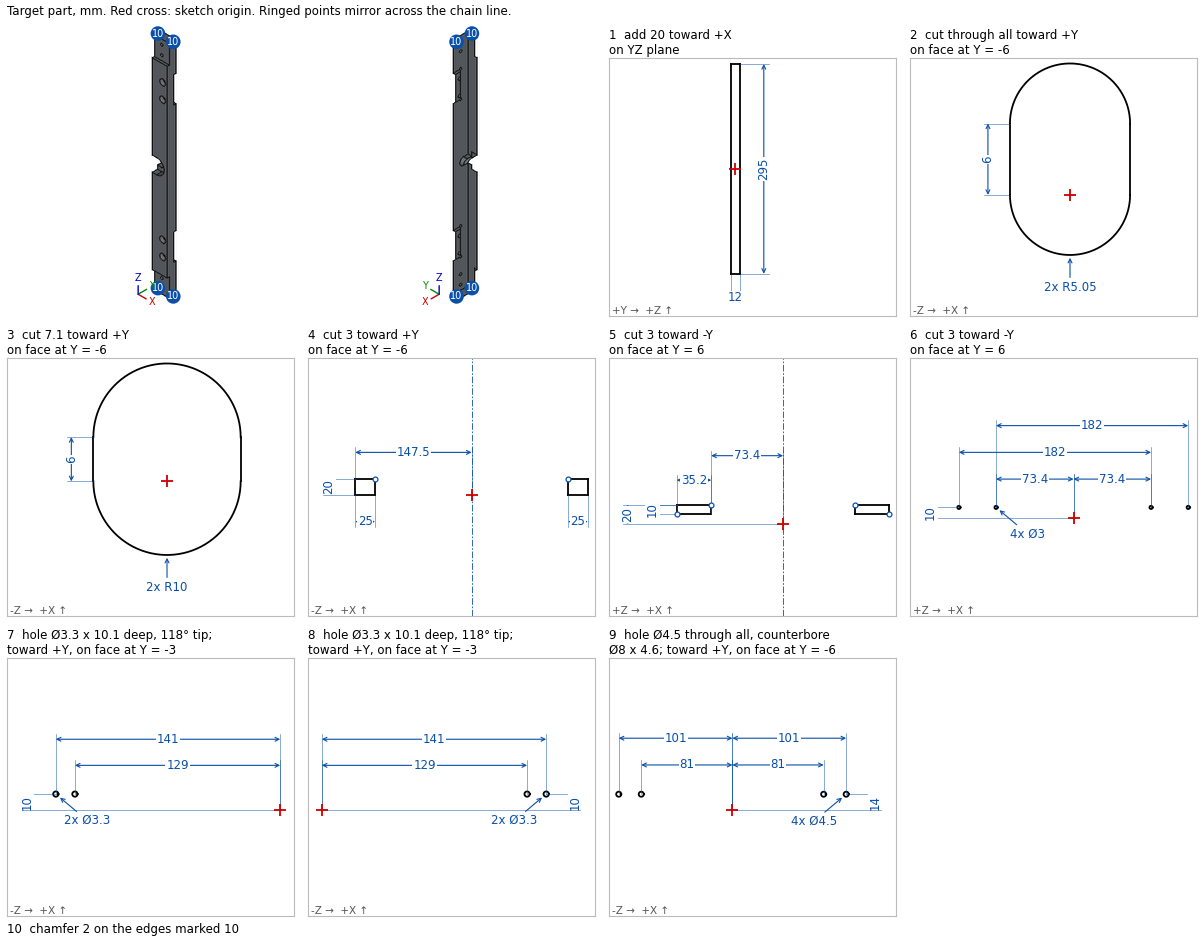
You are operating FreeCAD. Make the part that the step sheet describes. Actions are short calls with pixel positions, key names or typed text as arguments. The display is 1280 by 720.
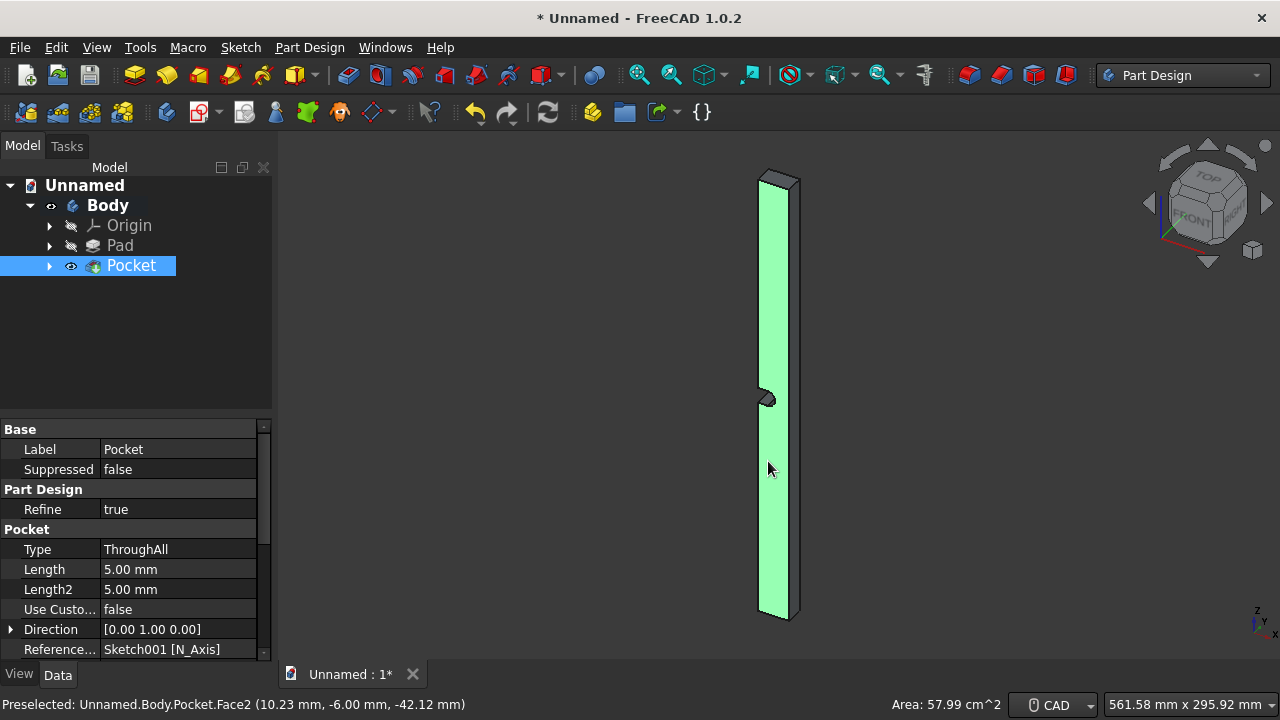
click(200, 112)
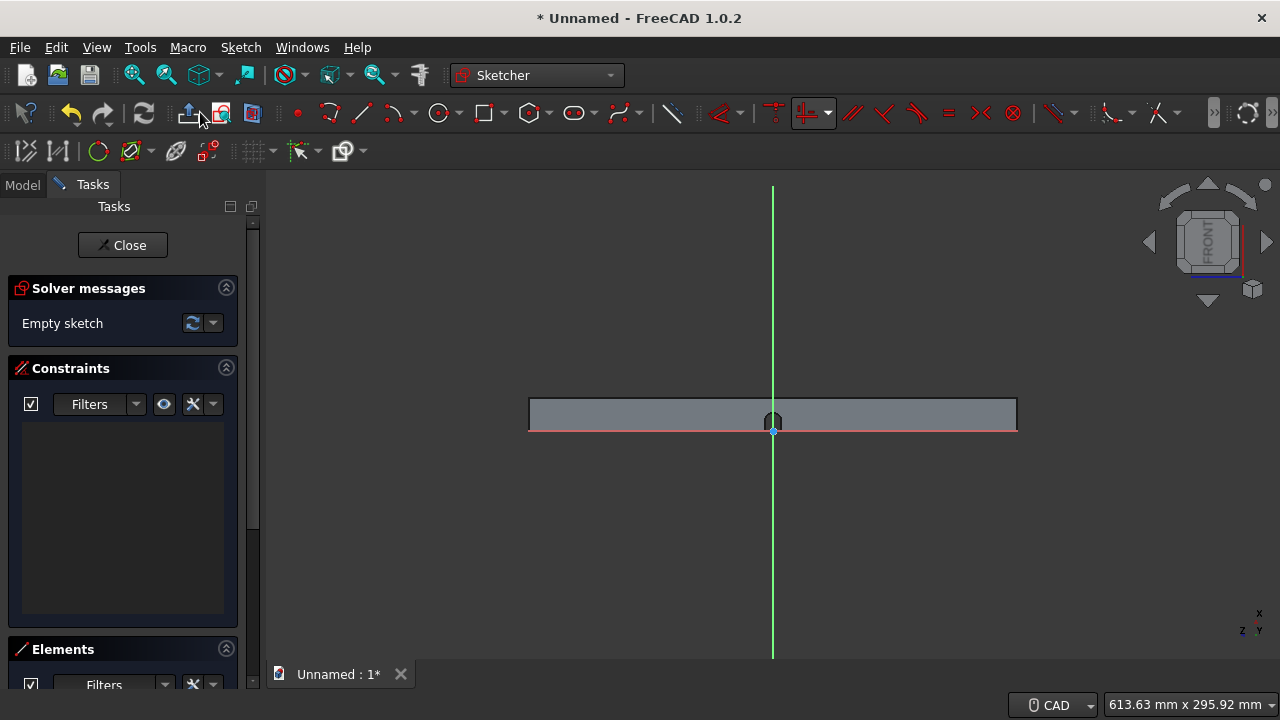
scroll(784, 428, up, 10)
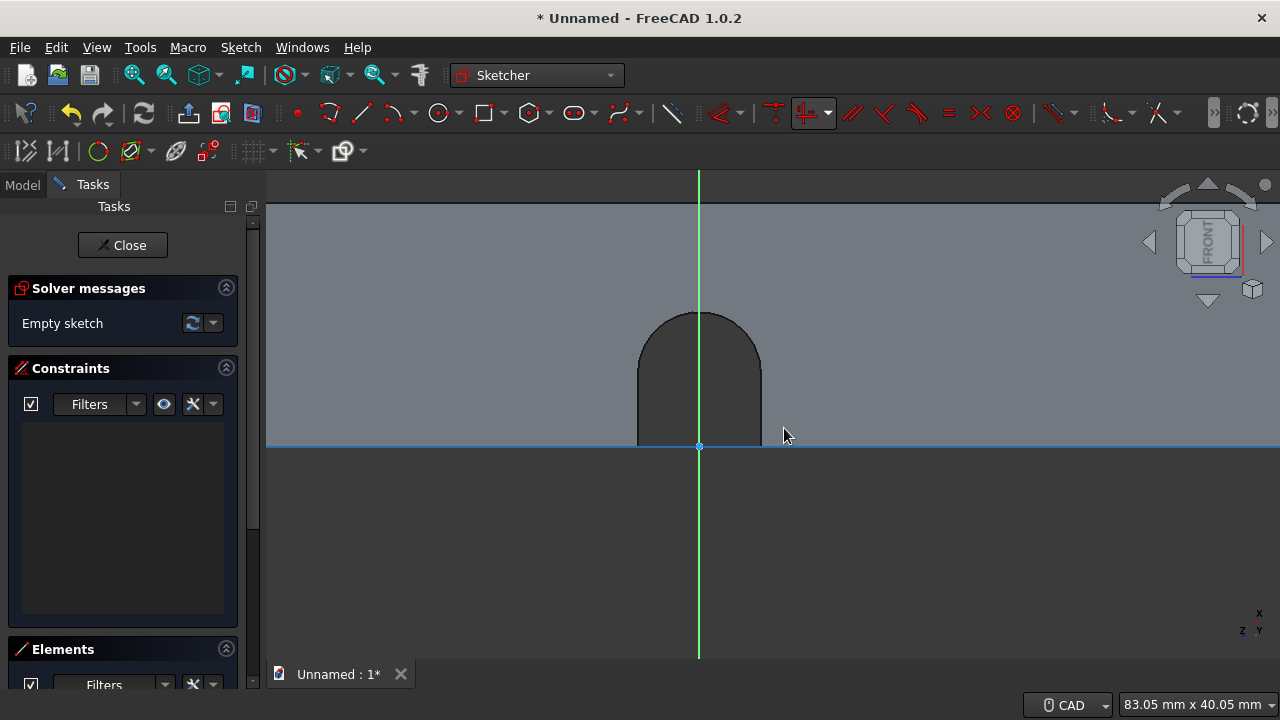
click(574, 114)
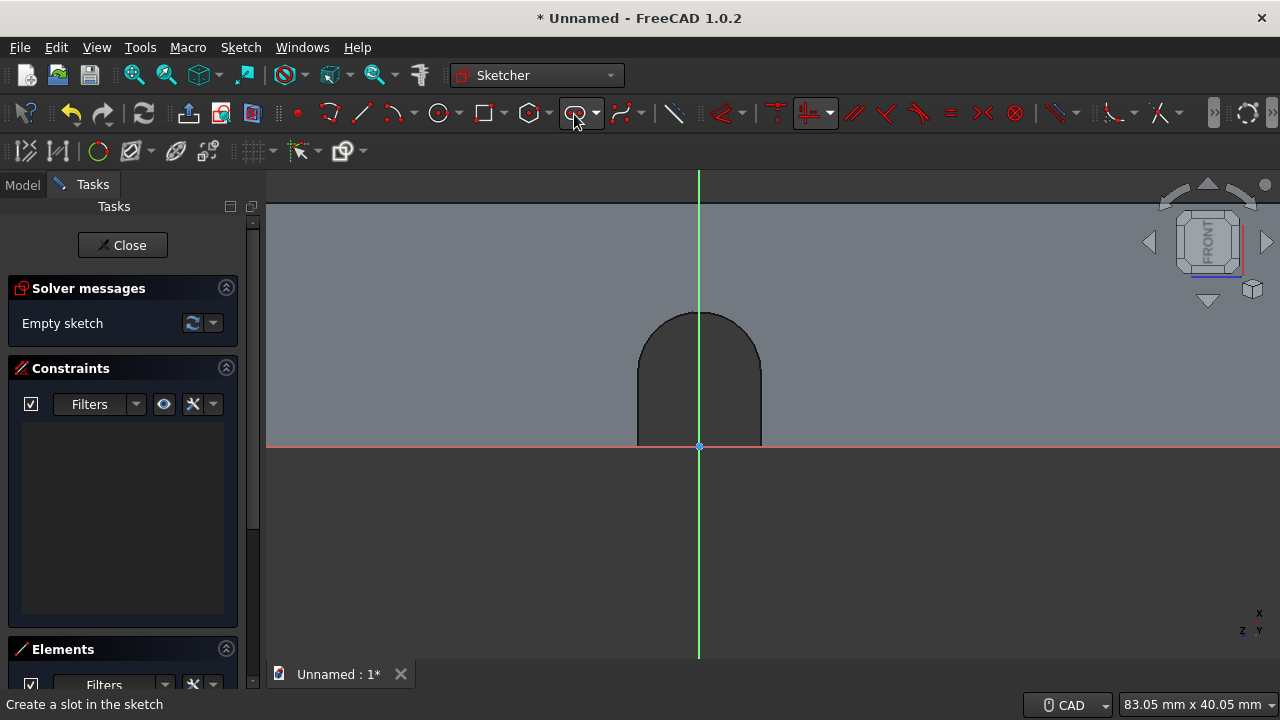
click(699, 447)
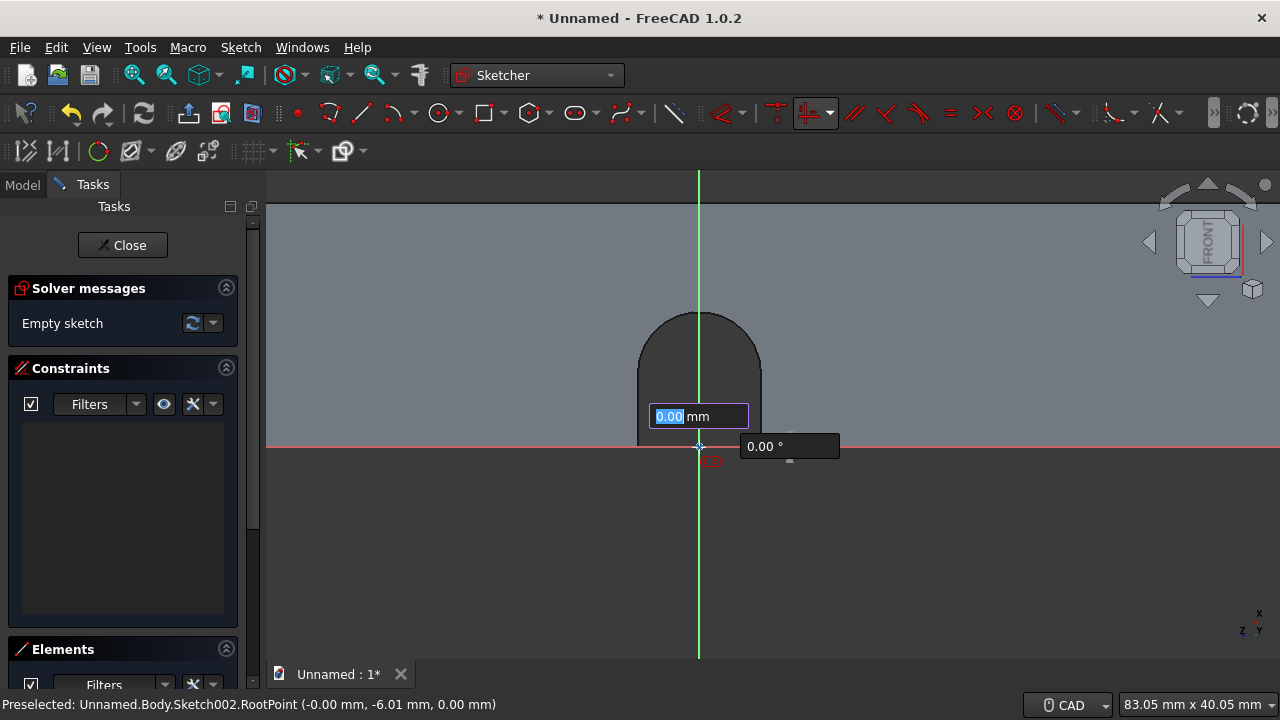
click(708, 374)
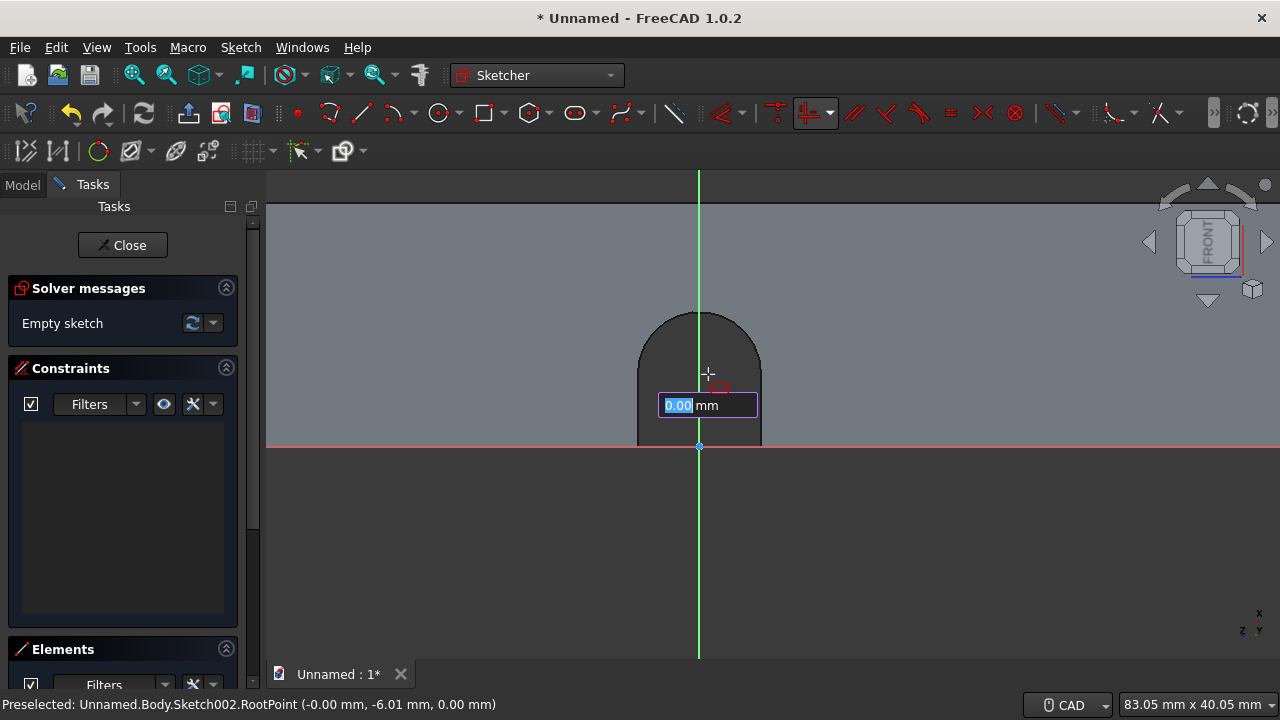
click(577, 410)
key(Escape)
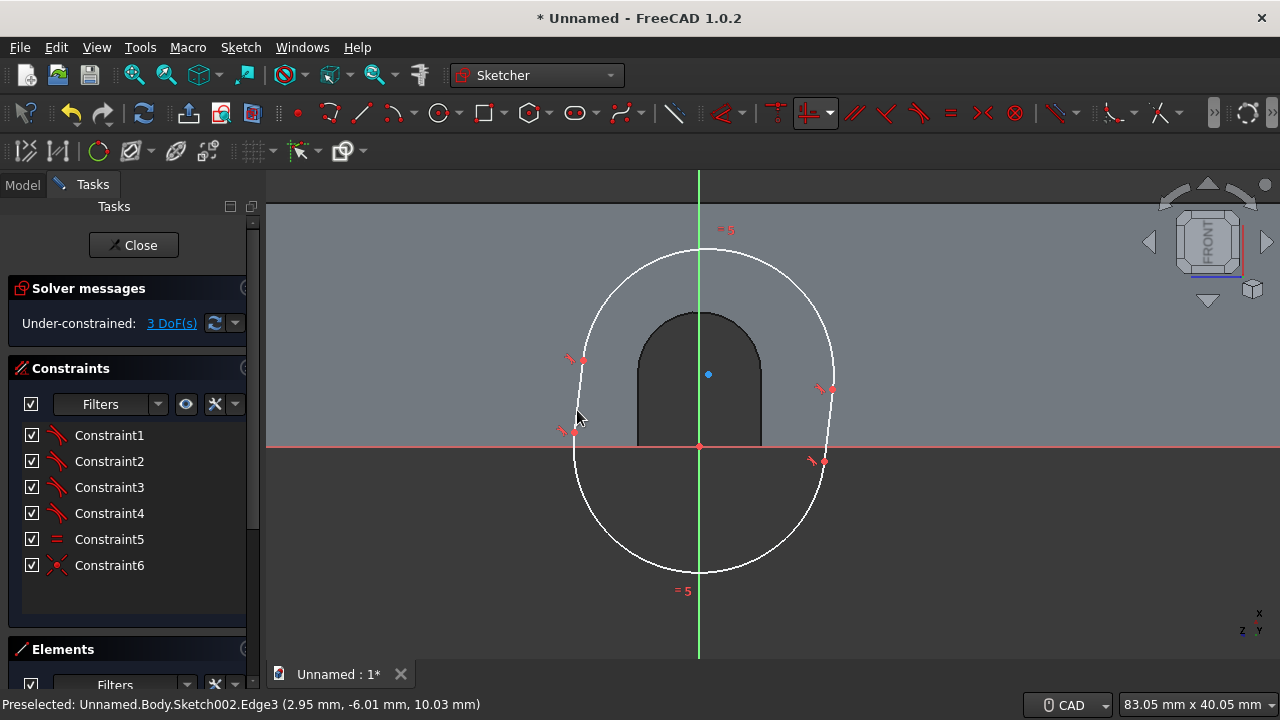
click(577, 411)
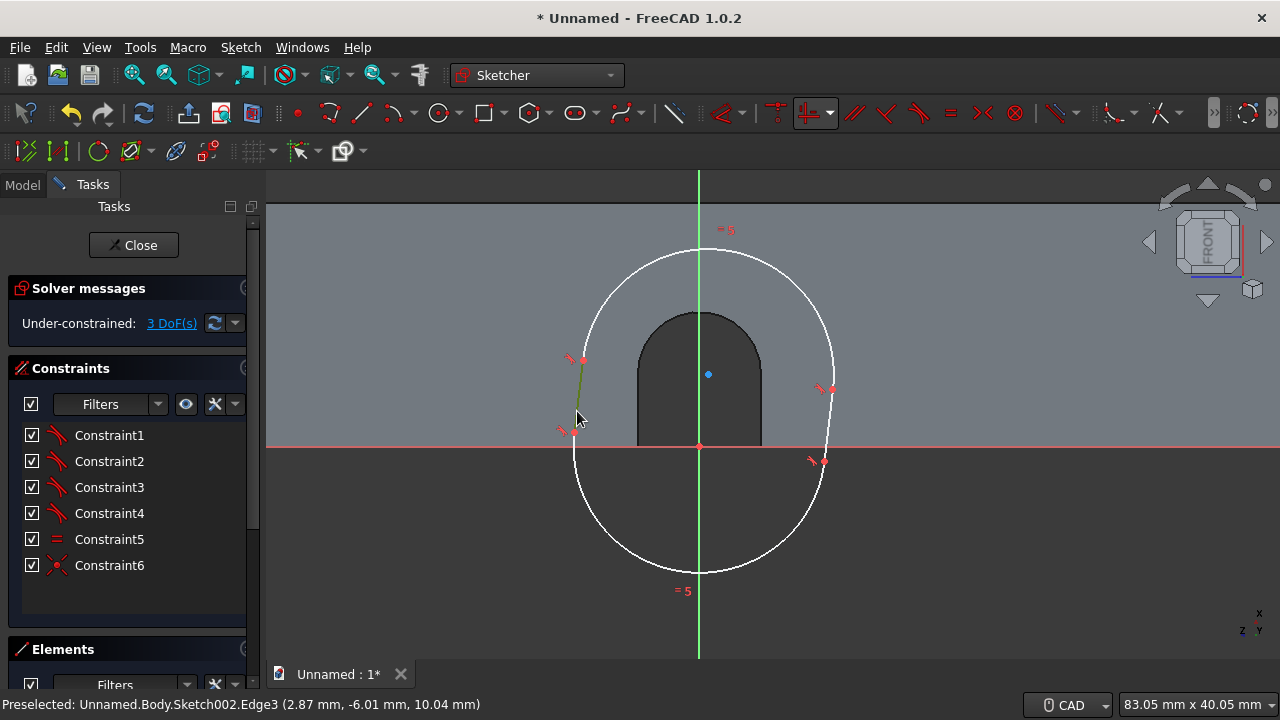
click(832, 114)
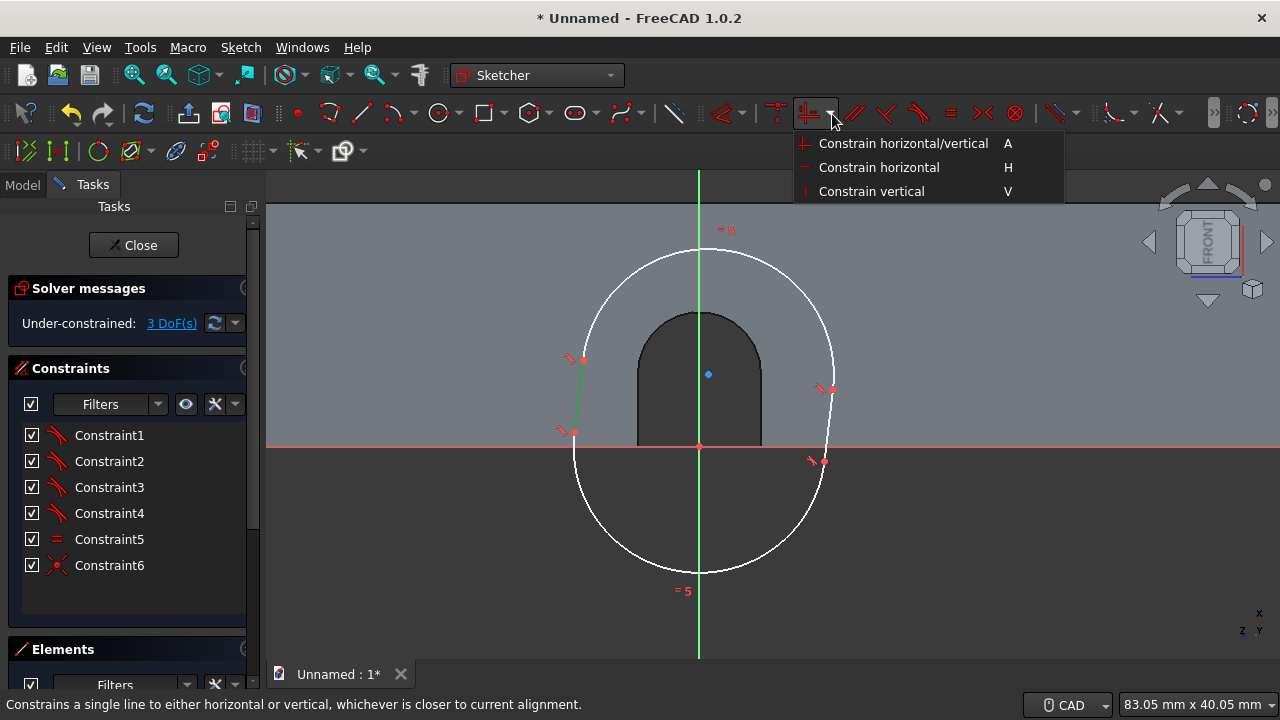
click(929, 191)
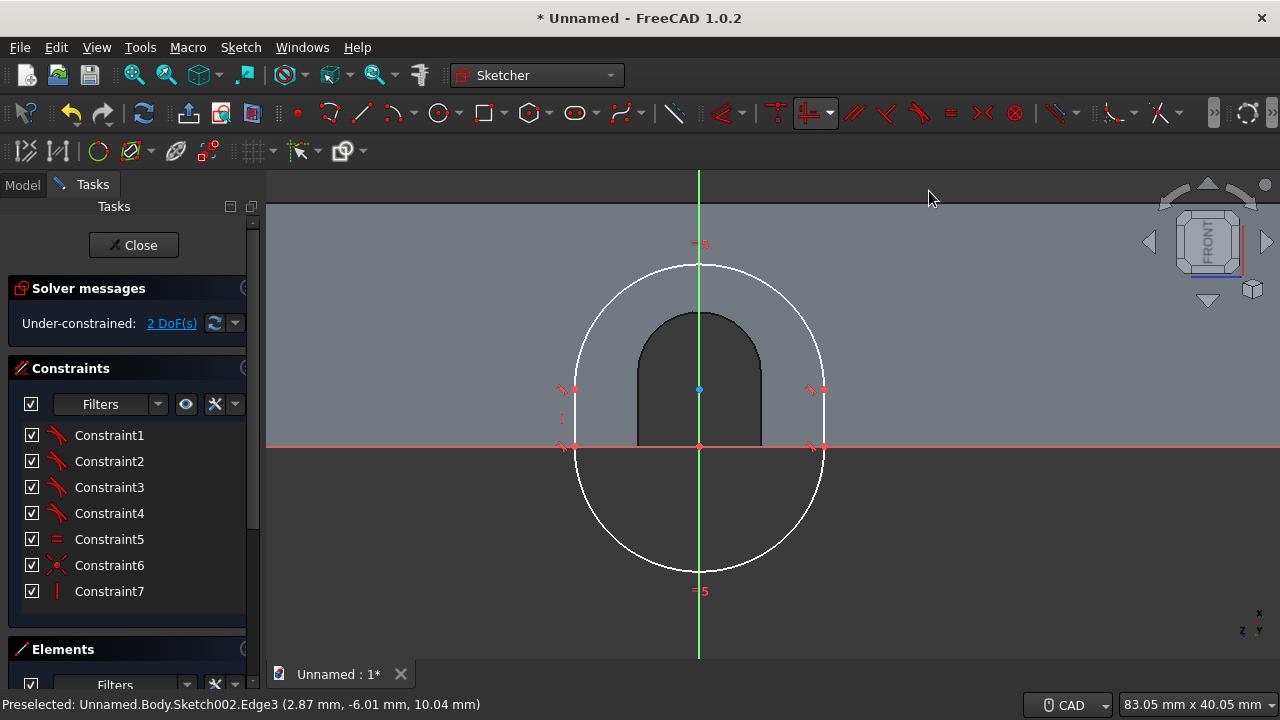
click(722, 114)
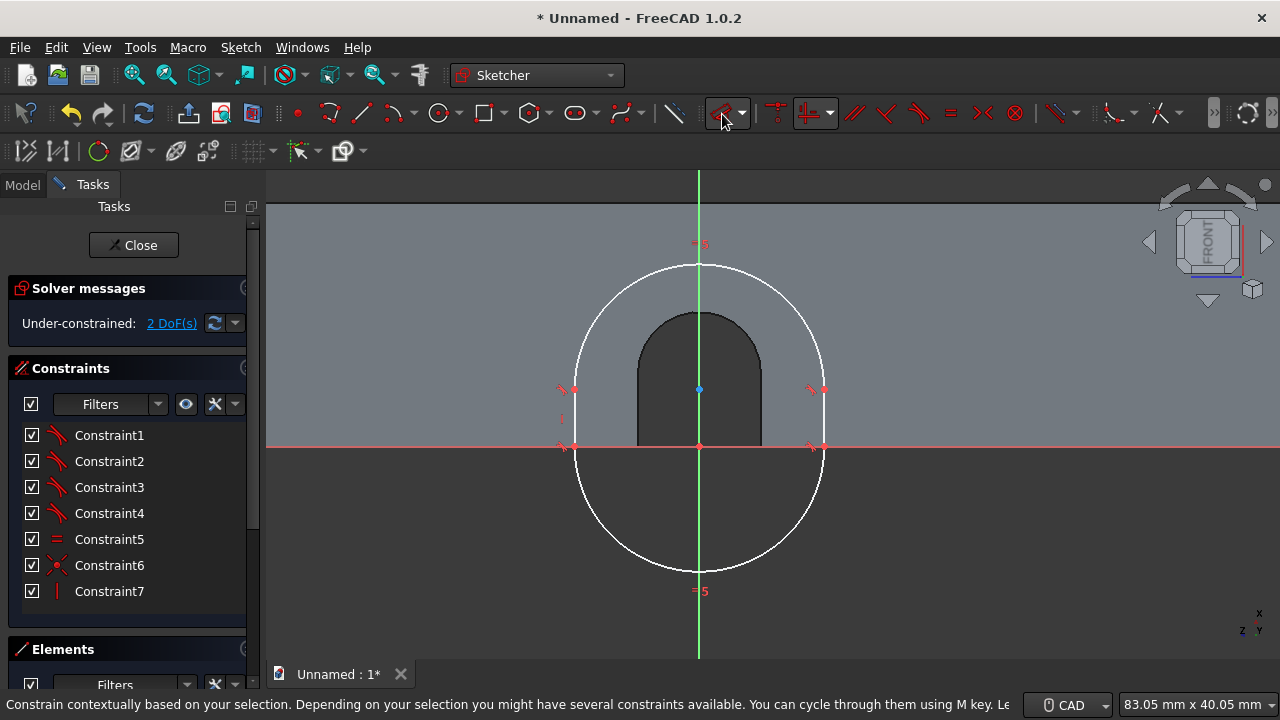
click(626, 548)
click(607, 574)